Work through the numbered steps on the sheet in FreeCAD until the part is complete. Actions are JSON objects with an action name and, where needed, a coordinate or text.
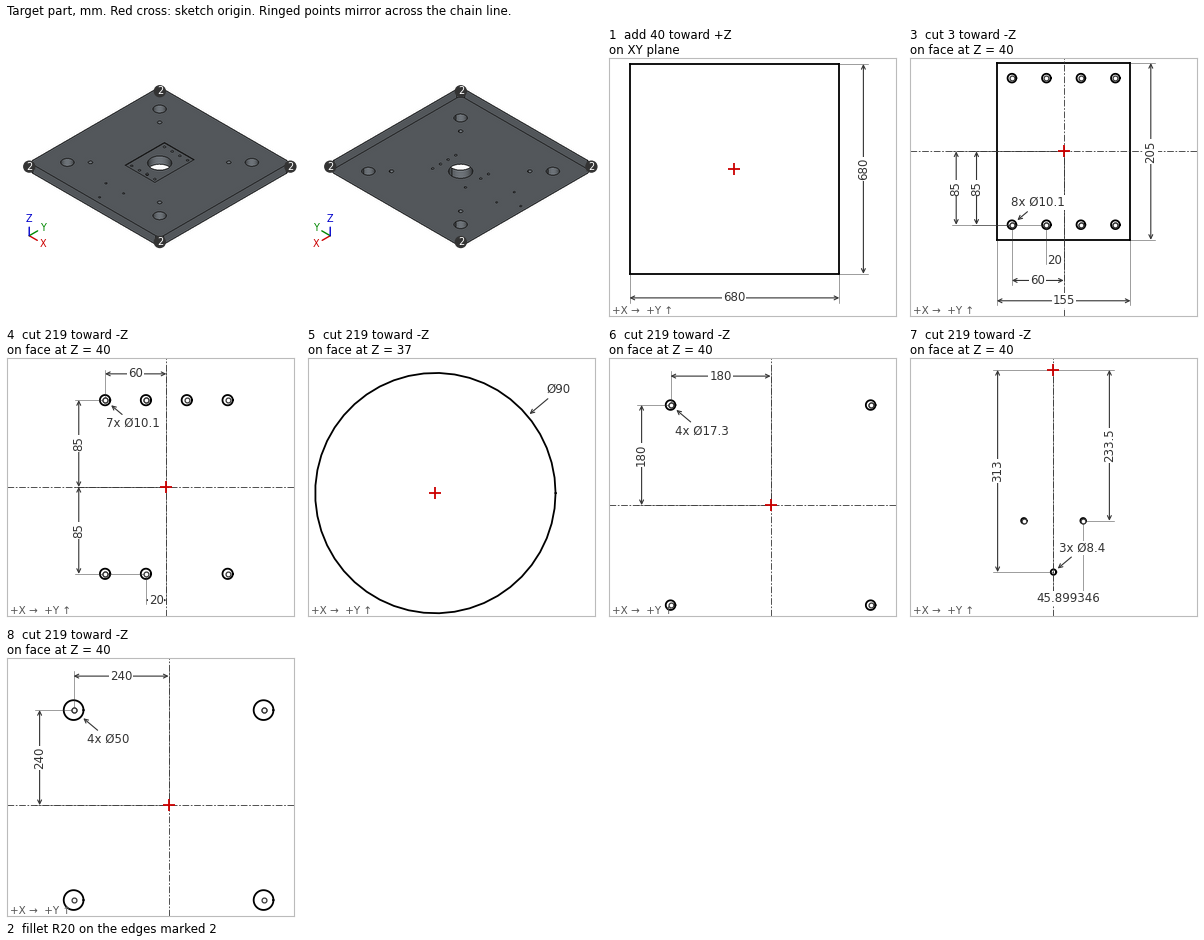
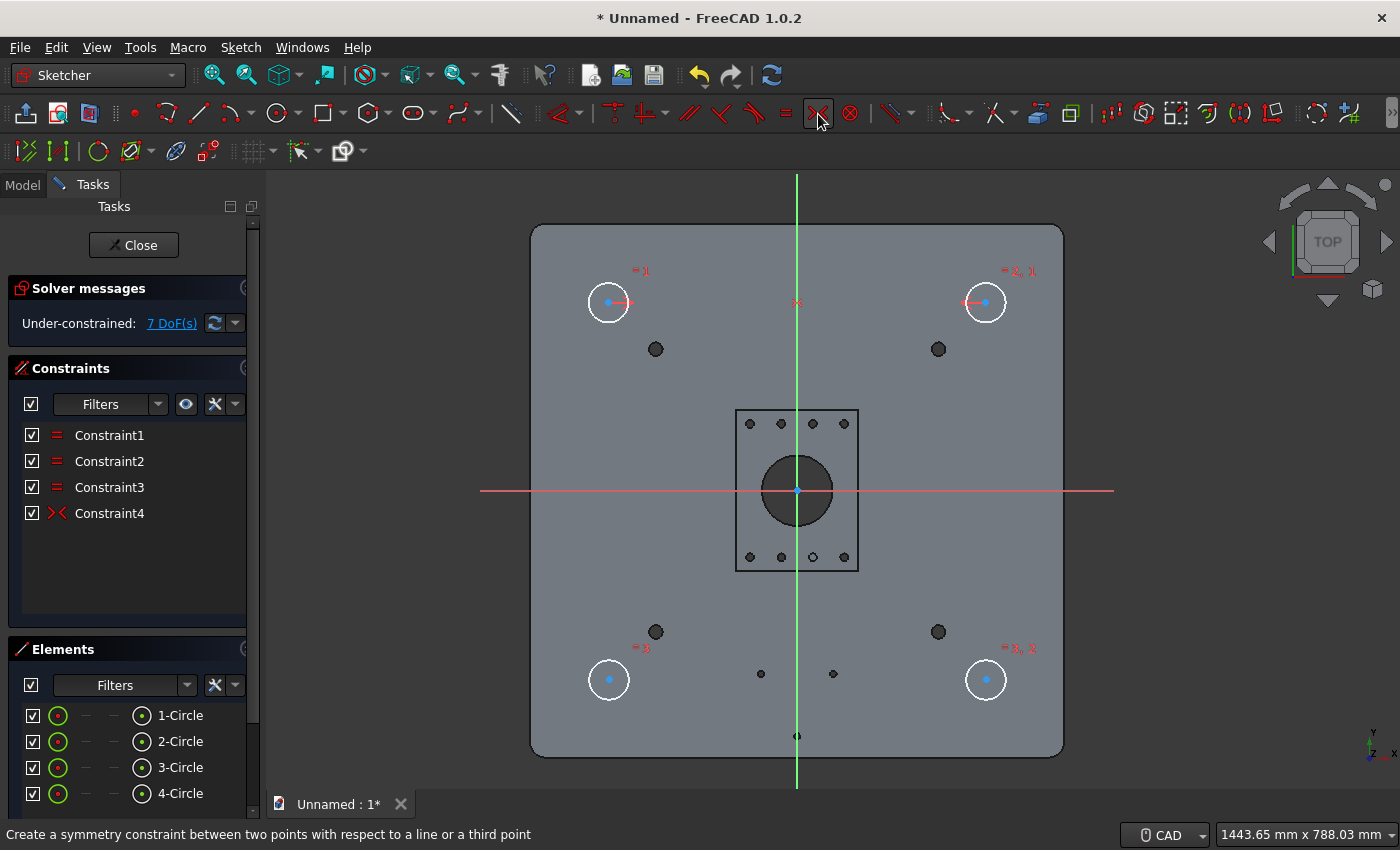
{"action": "left_click", "coordinate": [986, 303]}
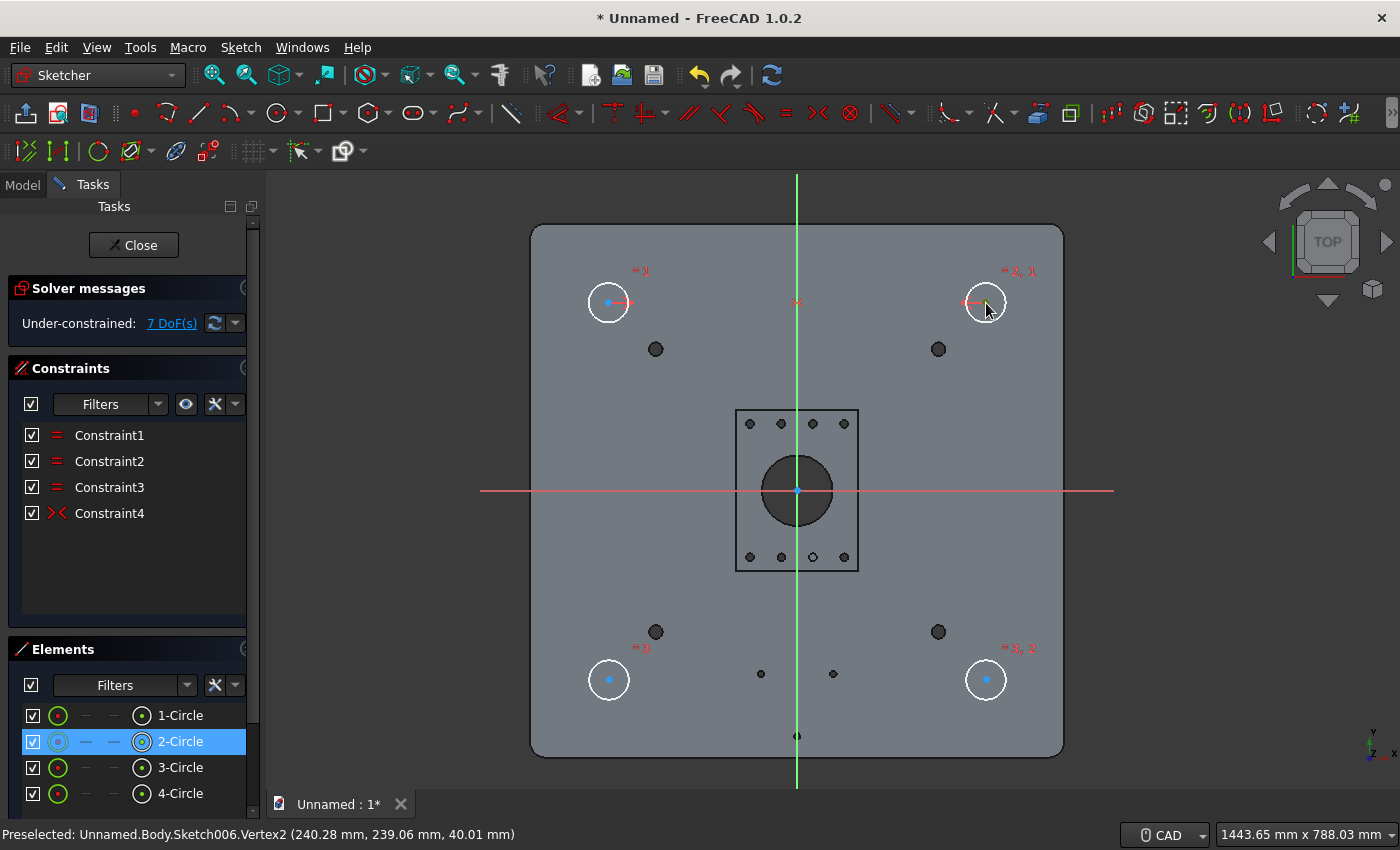
{"action": "left_click", "coordinate": [986, 680]}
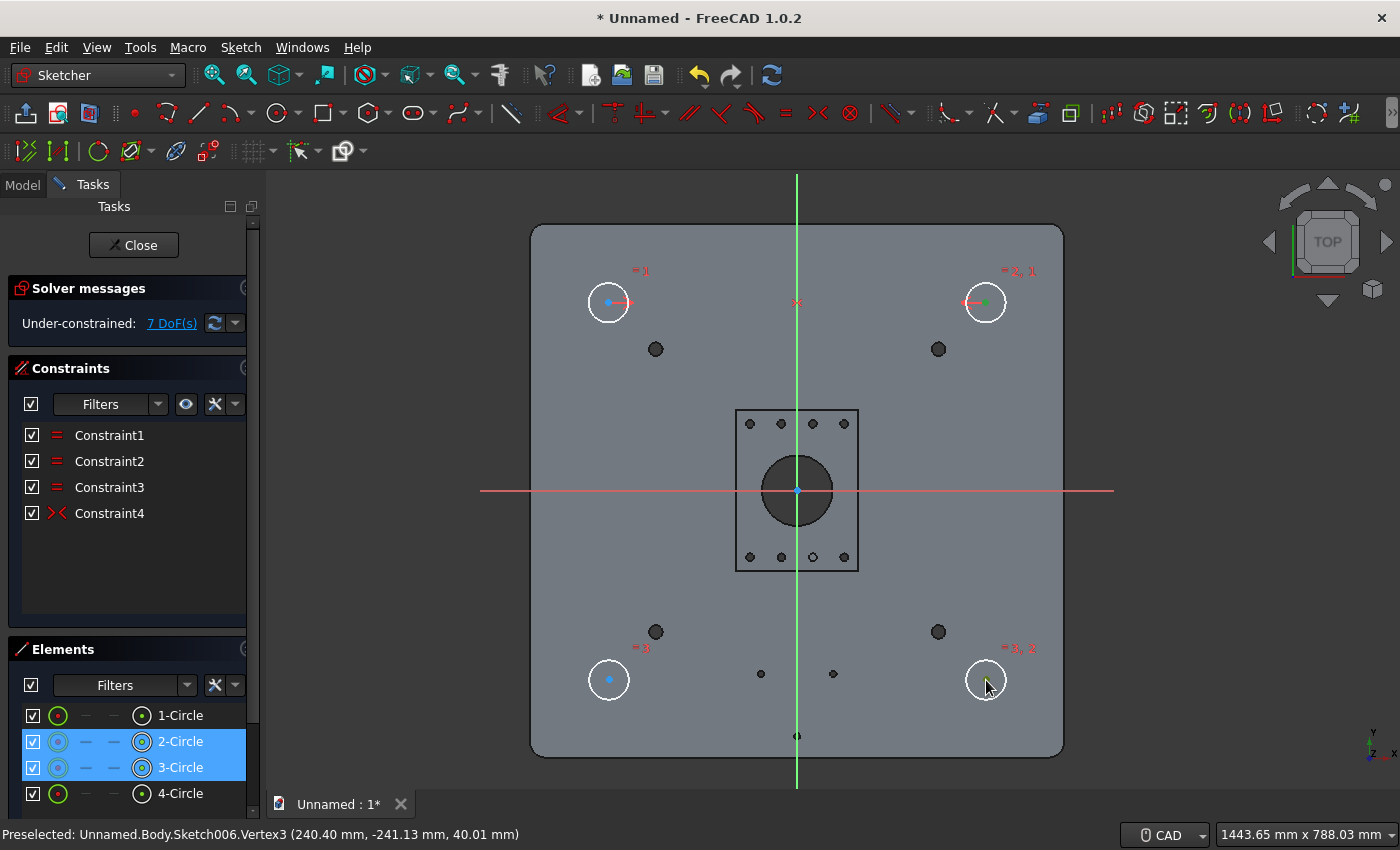
{"action": "left_click", "coordinate": [496, 491]}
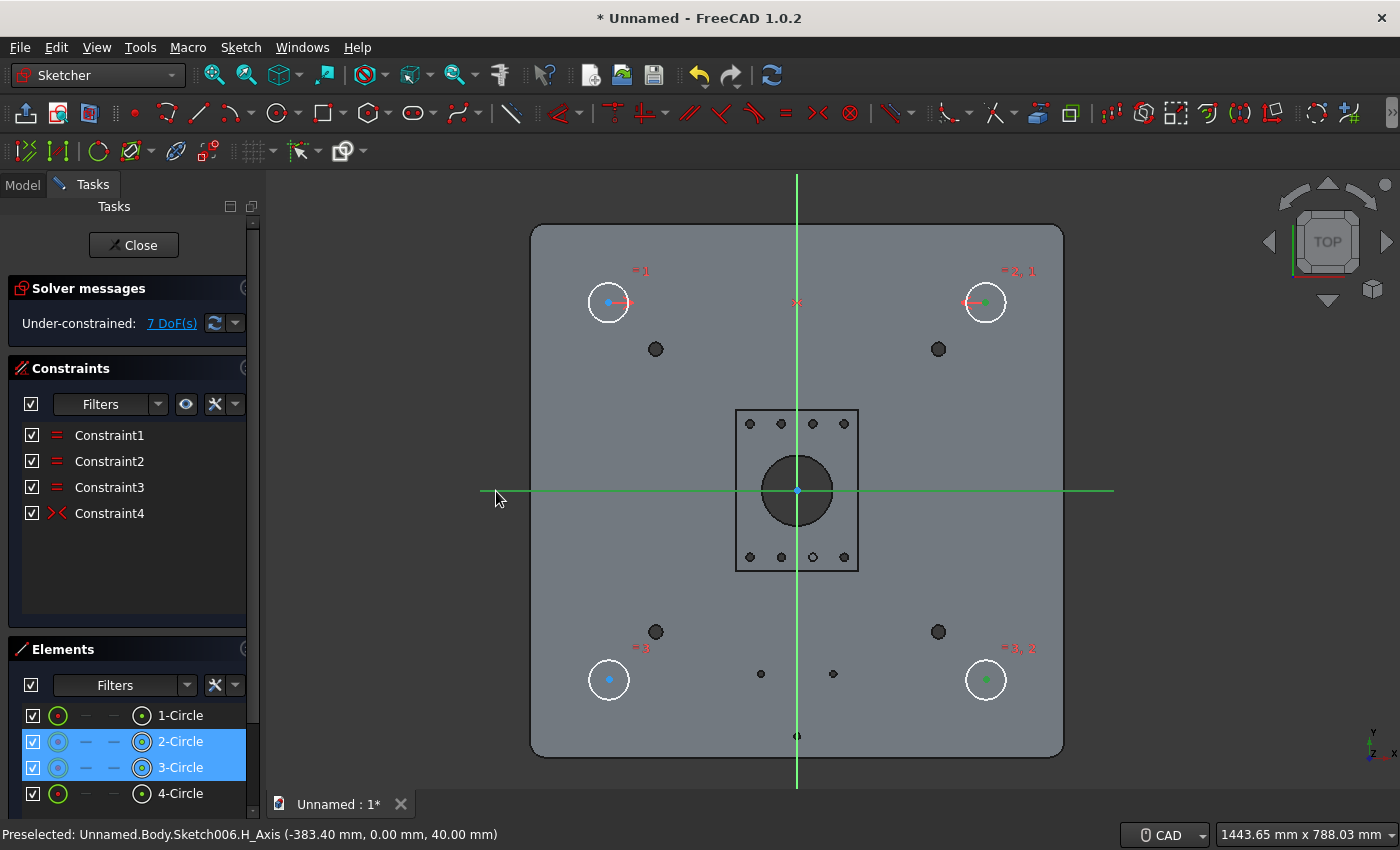
{"action": "left_click", "coordinate": [818, 114]}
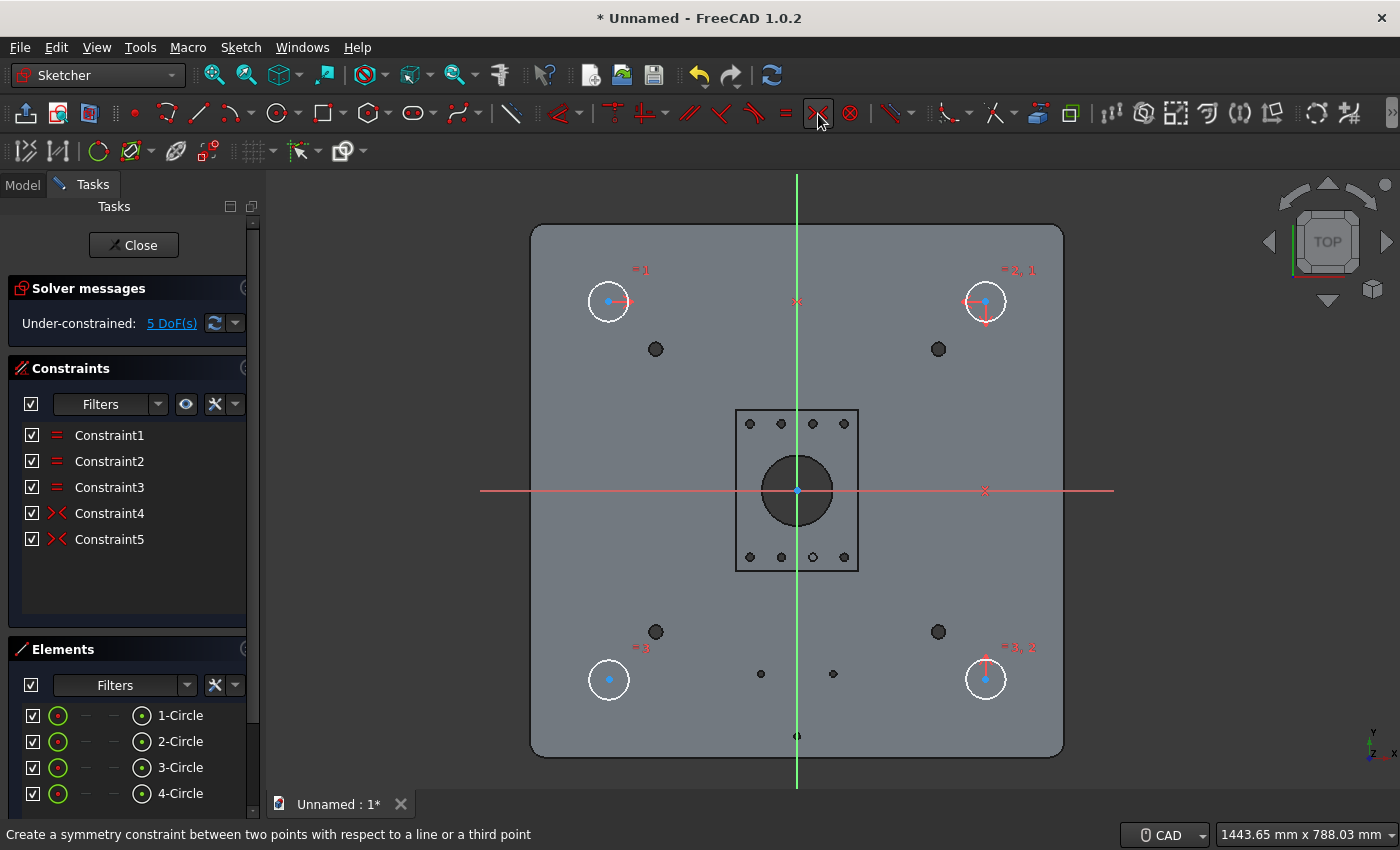
{"action": "left_click", "coordinate": [608, 302]}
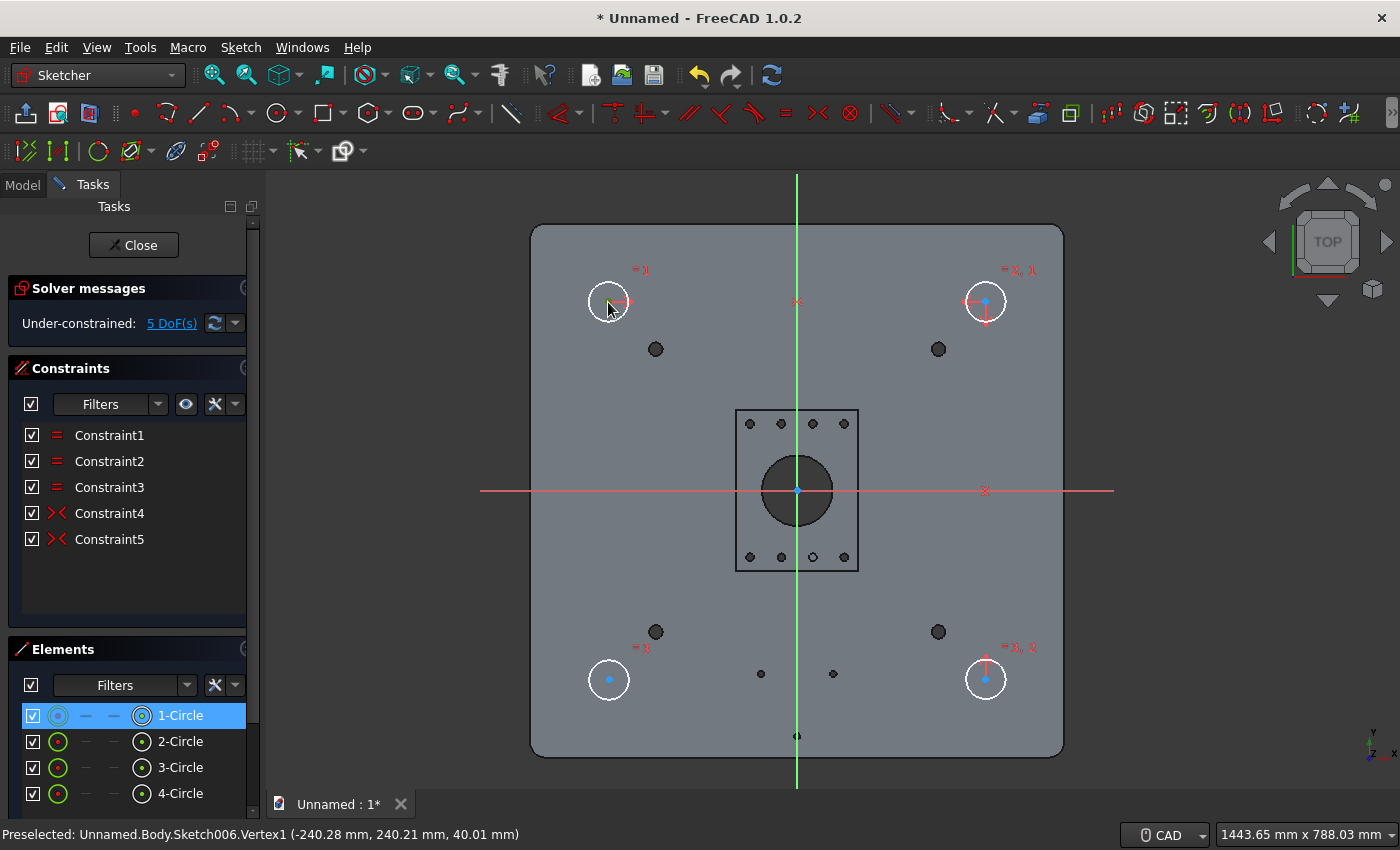
{"action": "left_click", "coordinate": [609, 680]}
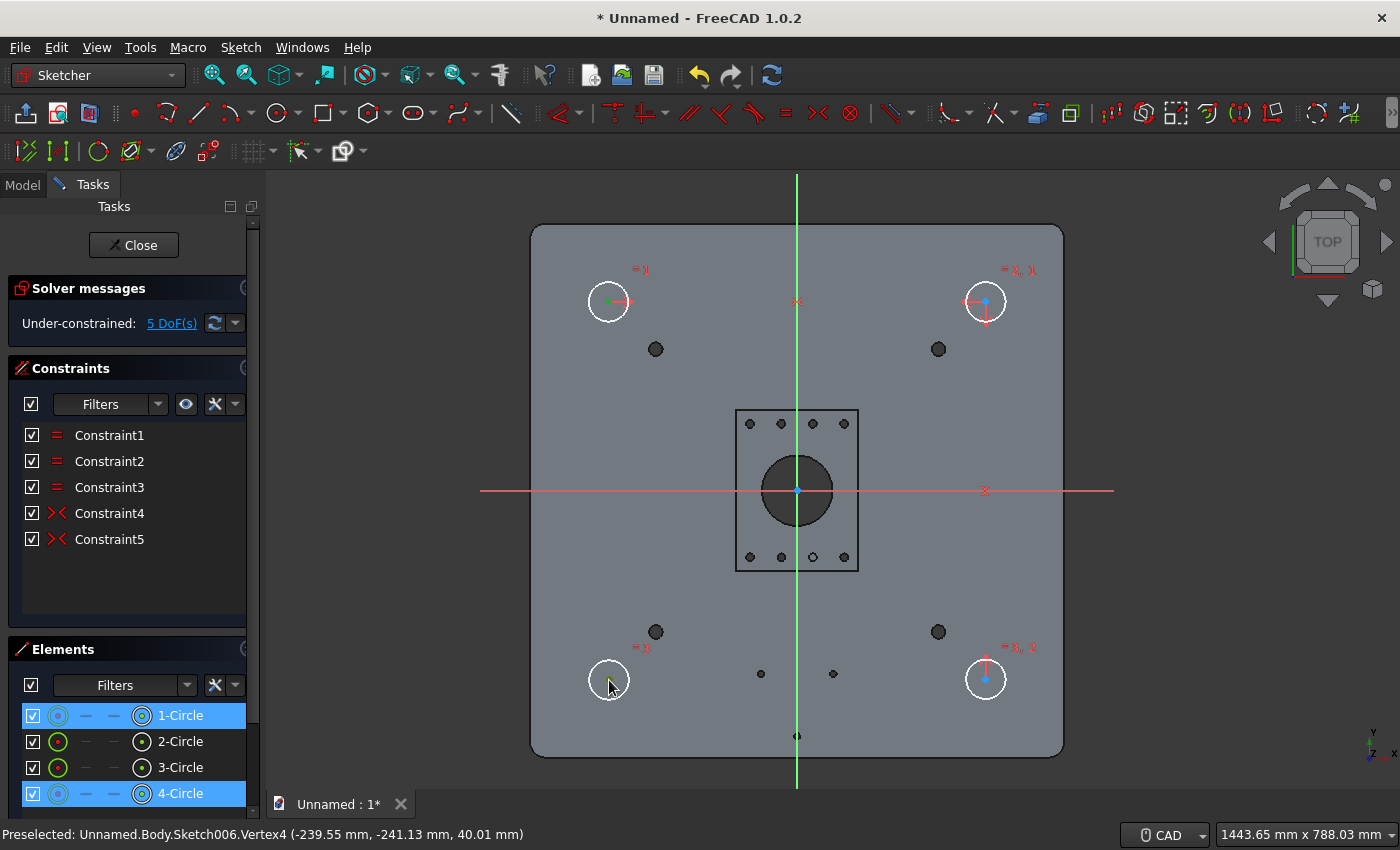
{"action": "left_click", "coordinate": [496, 491]}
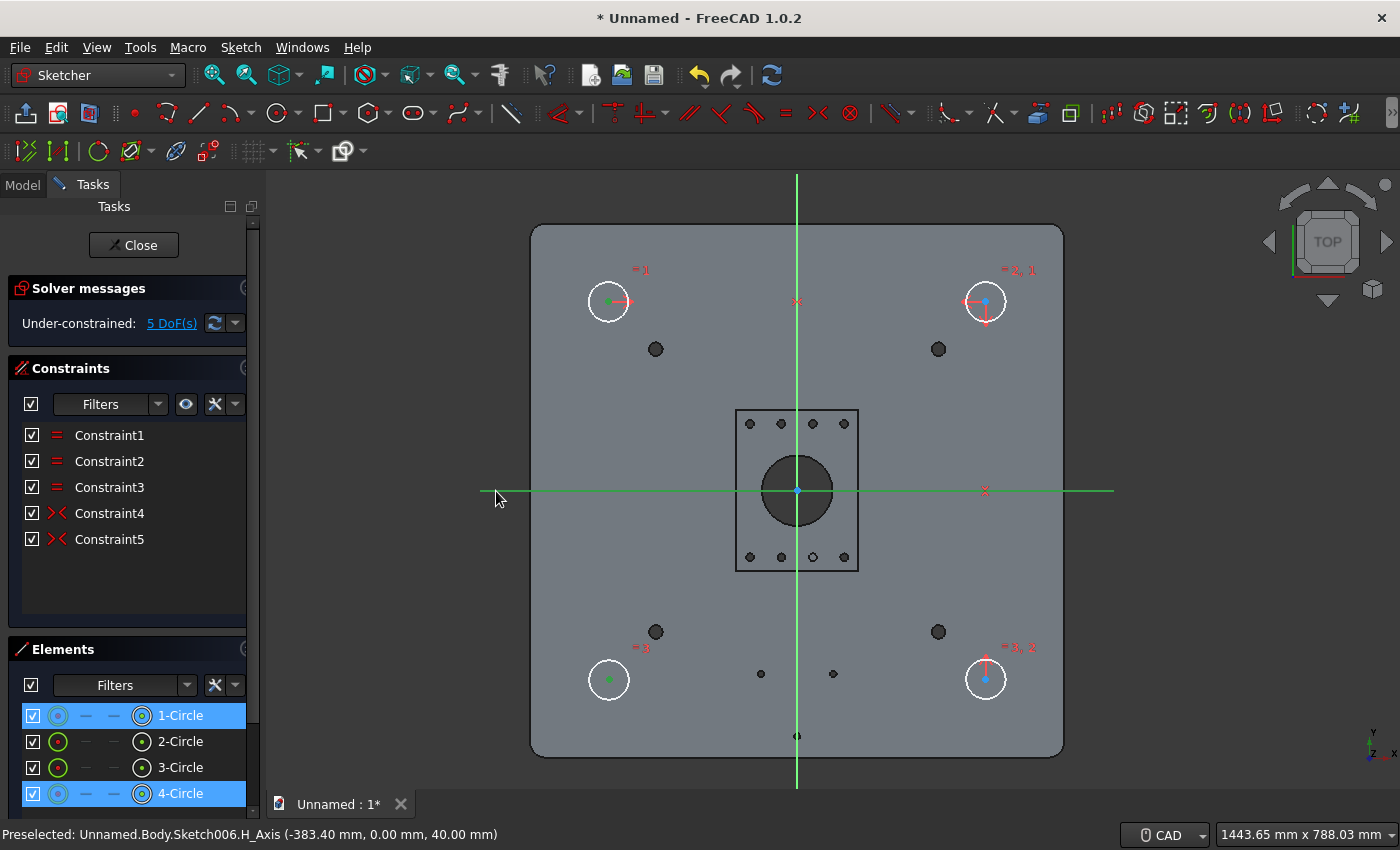
{"action": "left_click", "coordinate": [818, 114]}